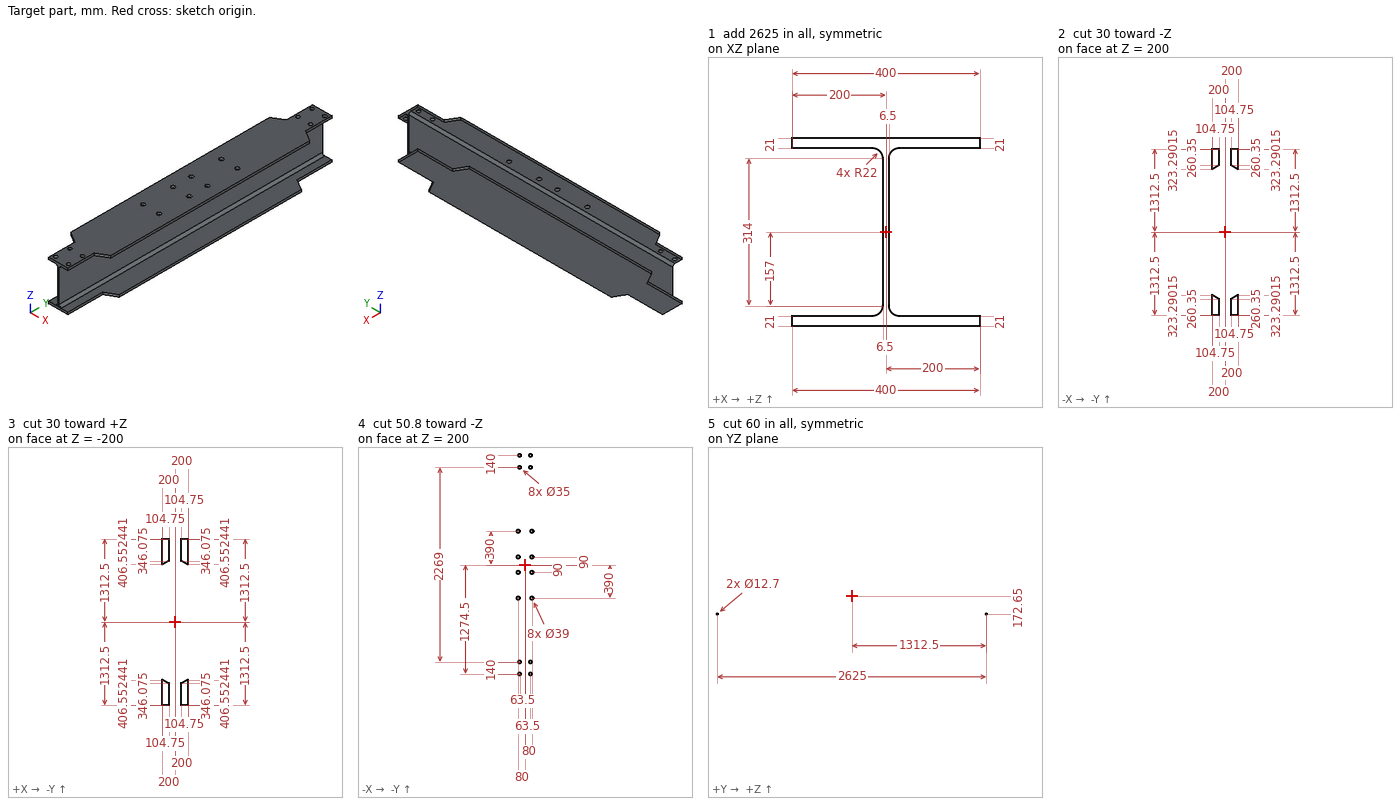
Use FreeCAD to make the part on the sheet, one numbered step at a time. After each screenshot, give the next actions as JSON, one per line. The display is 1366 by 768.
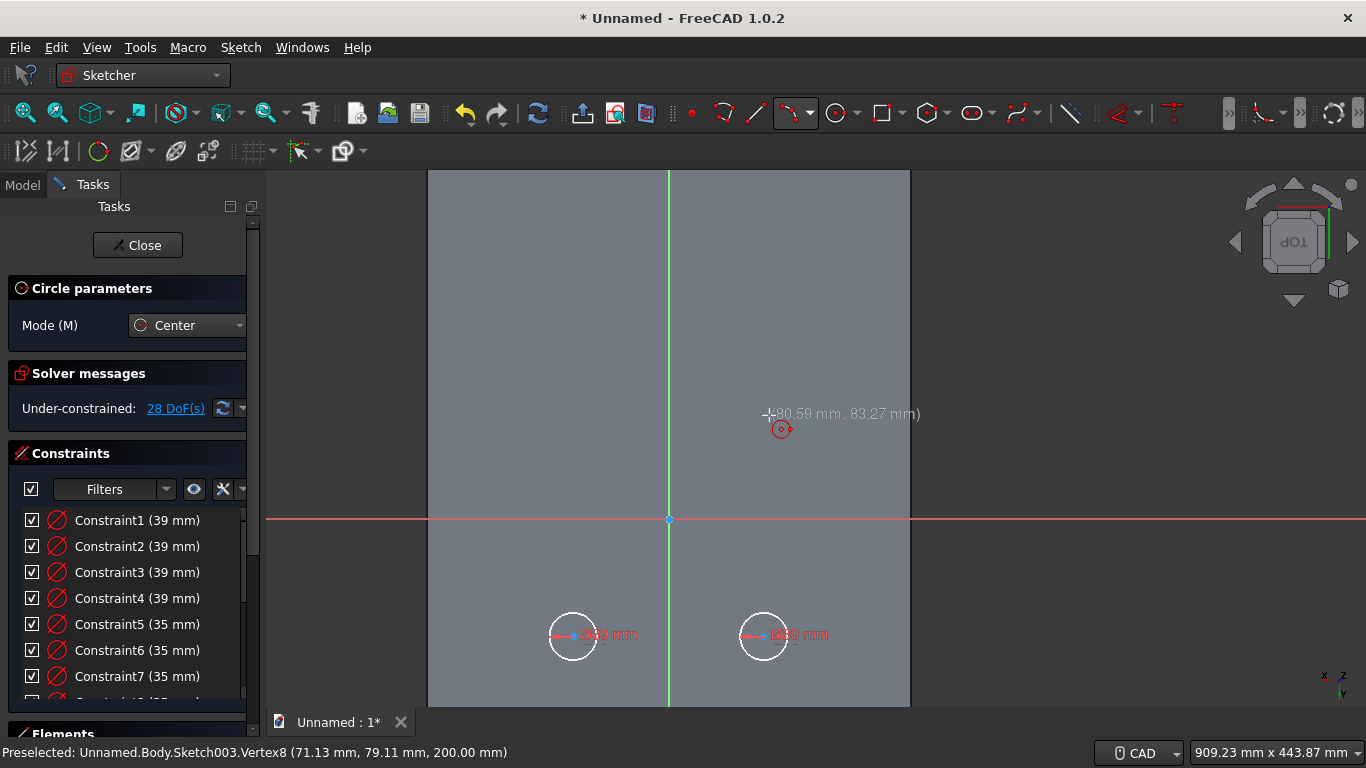
{"action": "scroll", "coordinate": [757, 428], "scroll_direction": "down", "scroll_amount": 11}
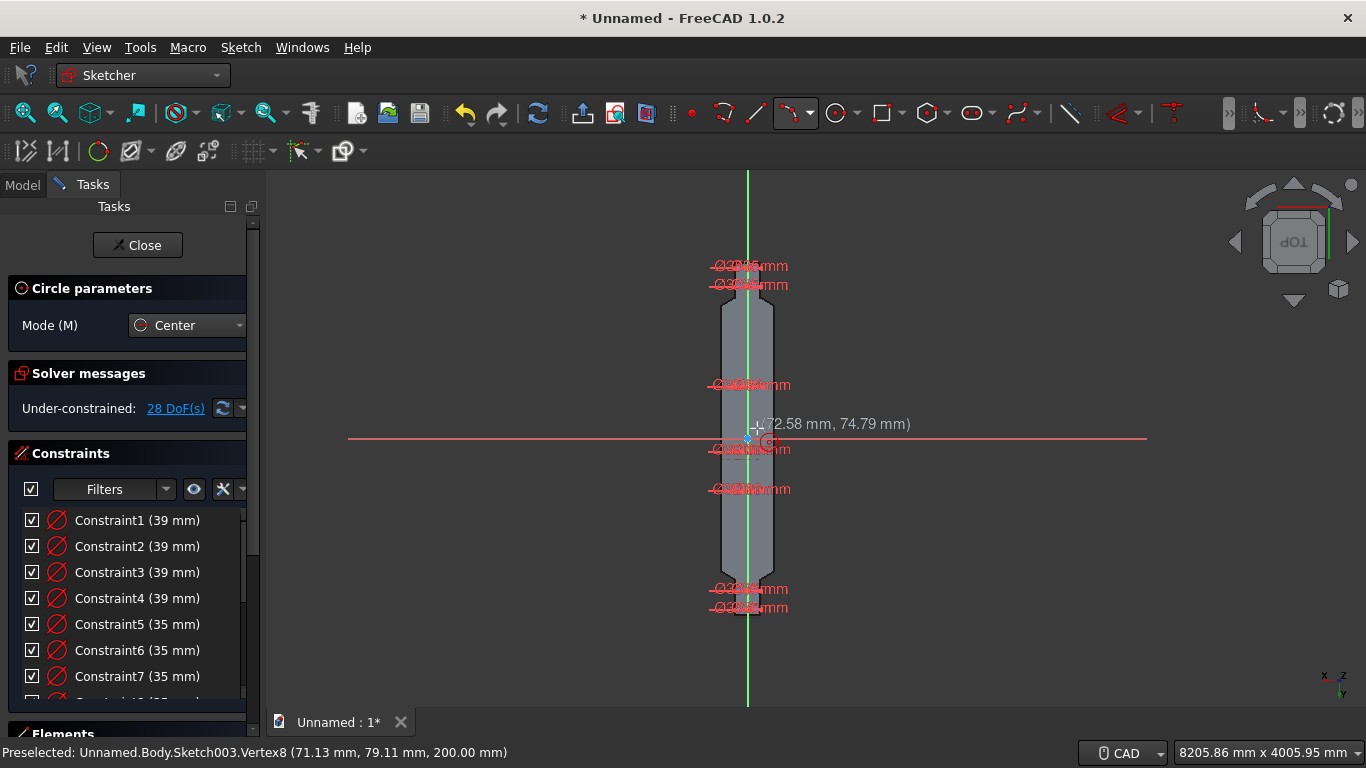
{"action": "scroll", "coordinate": [758, 426], "scroll_direction": "up", "scroll_amount": 2}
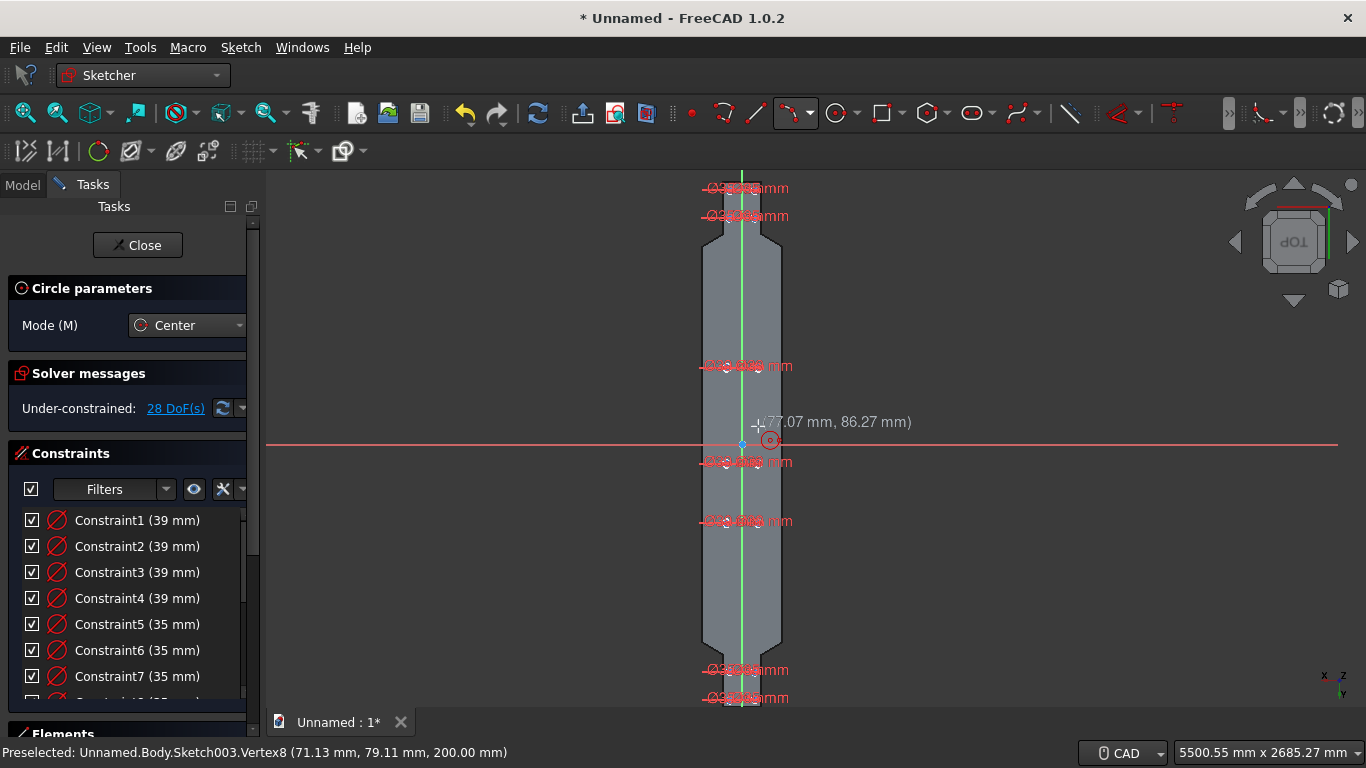
{"action": "left_click", "coordinate": [758, 427]}
{"action": "mouse_move", "coordinate": [761, 424]}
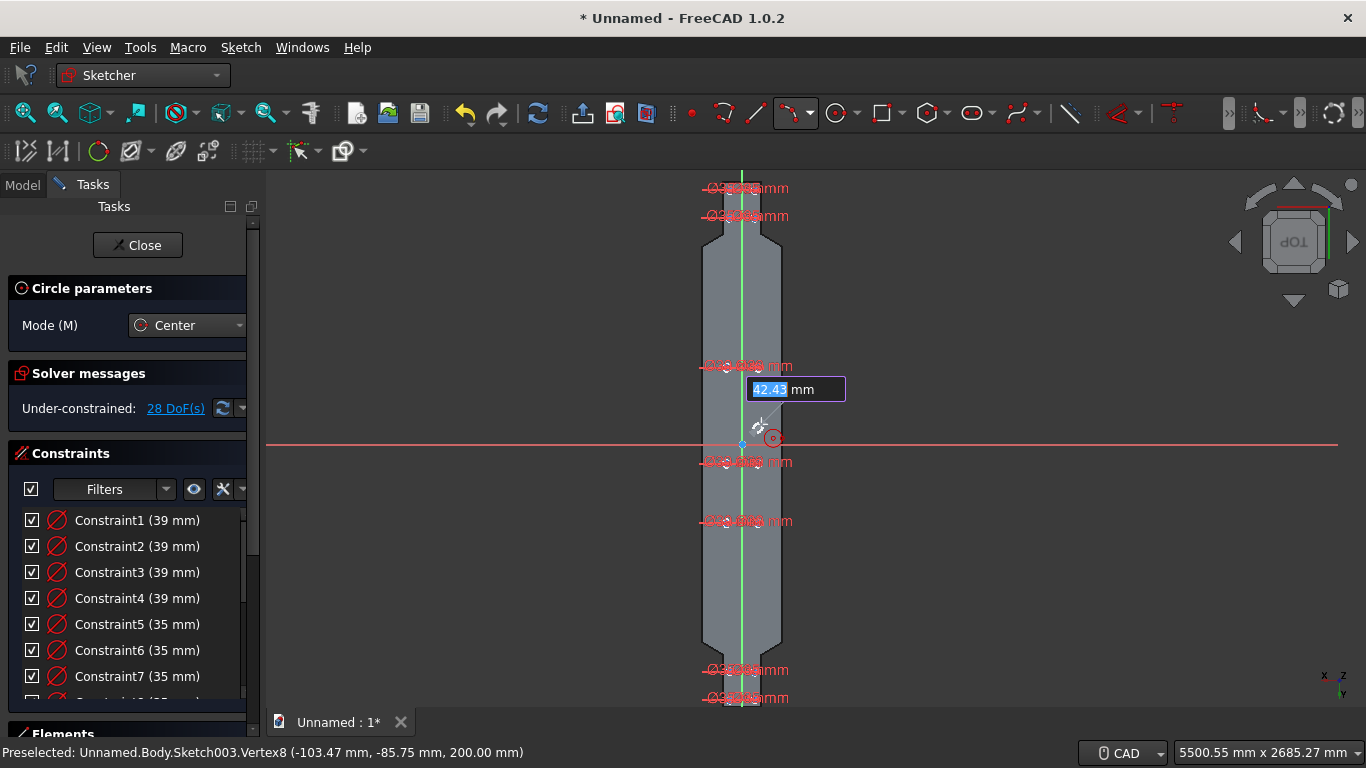
{"action": "type", "text": "39"}
{"action": "key", "text": "Return"}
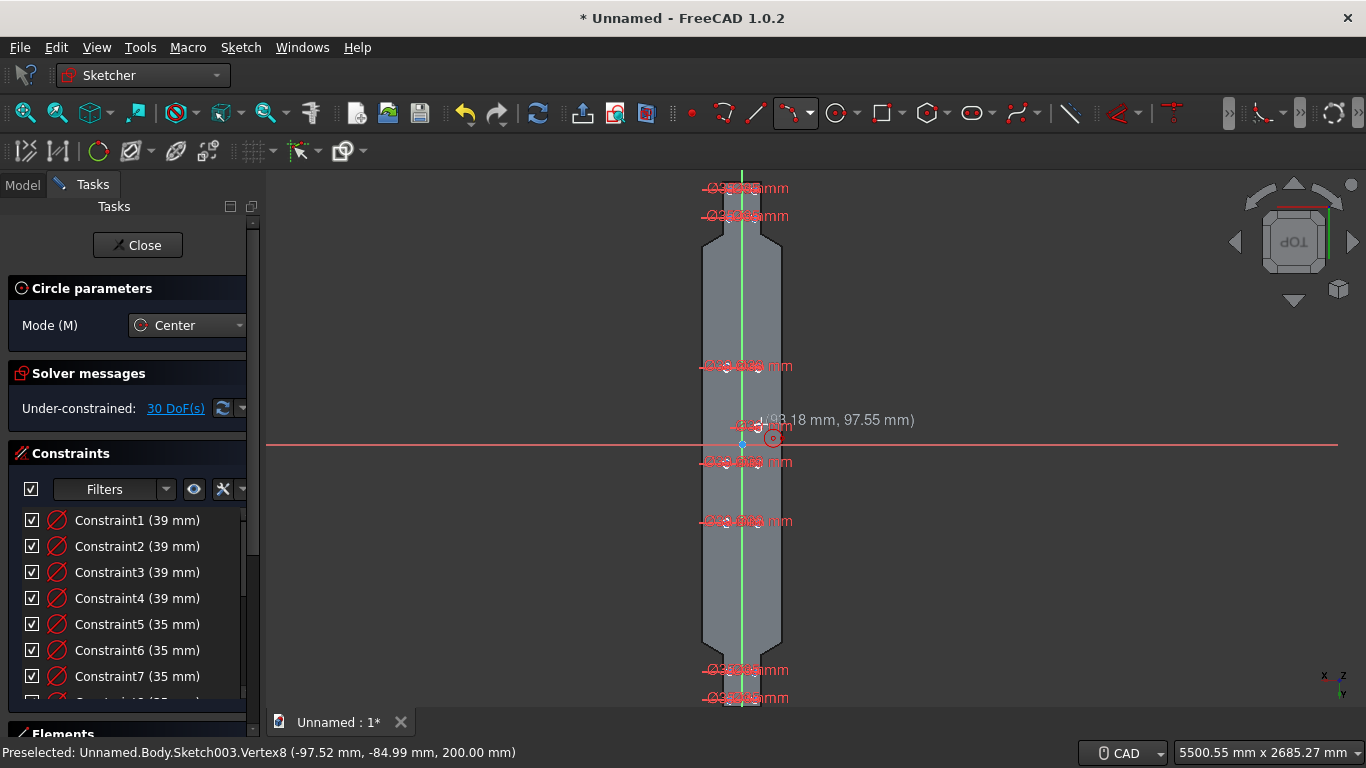
{"action": "scroll", "coordinate": [726, 427], "scroll_direction": "up", "scroll_amount": 9}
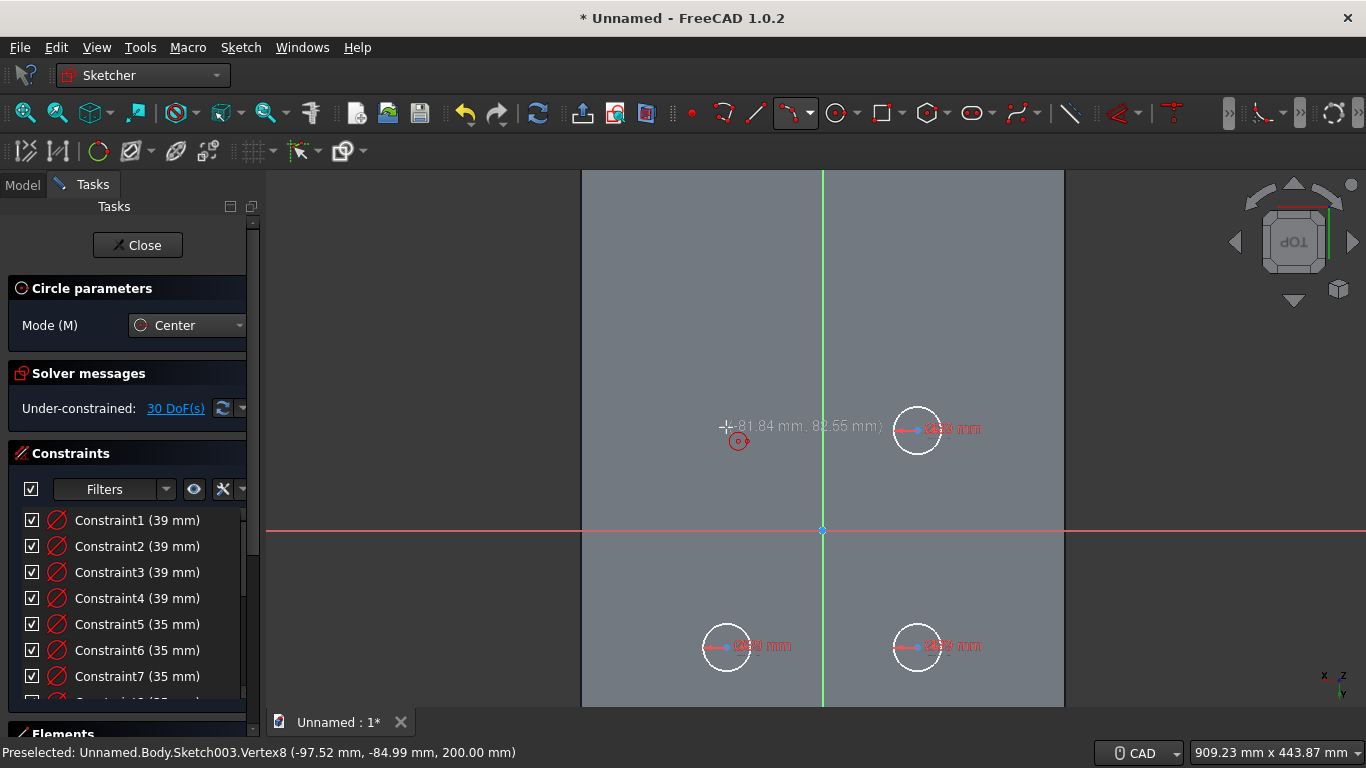
{"action": "scroll", "coordinate": [738, 427], "scroll_direction": "down", "scroll_amount": 11}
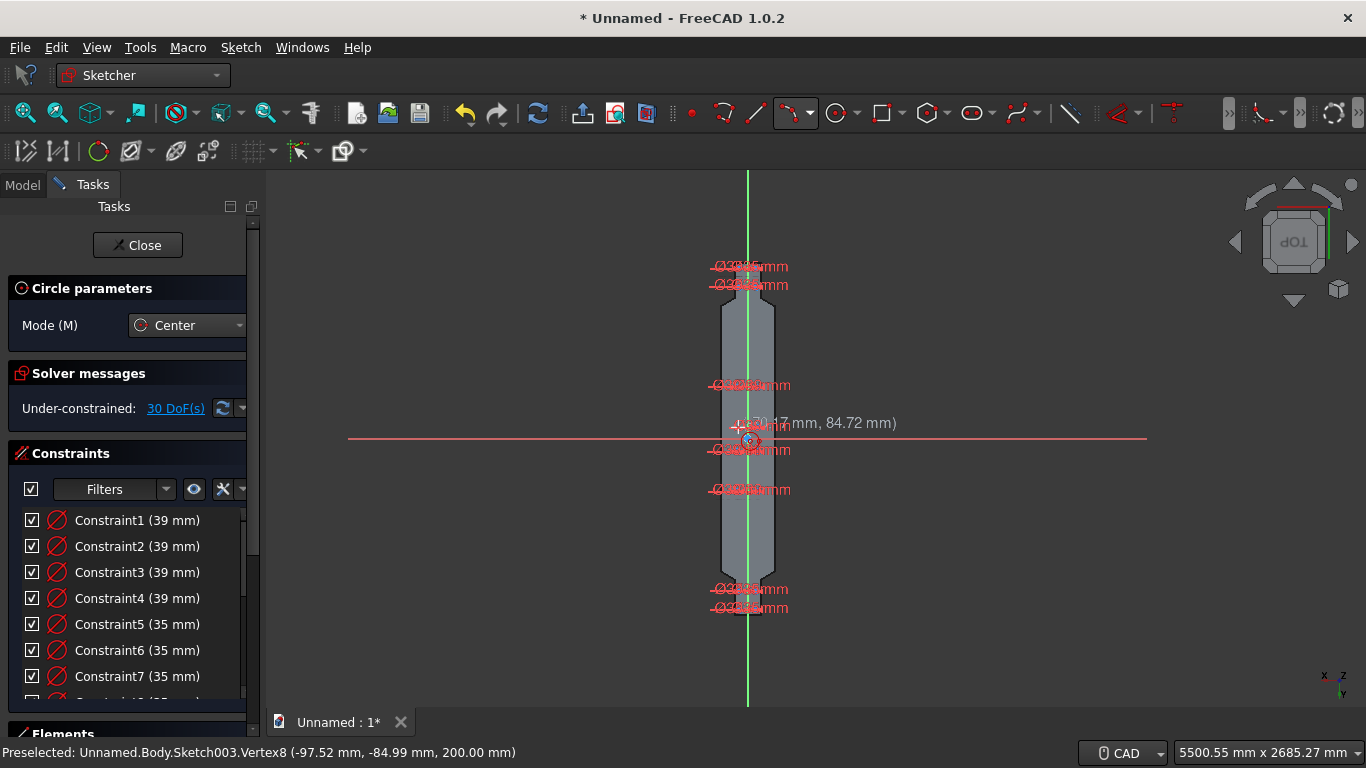
{"action": "scroll", "coordinate": [737, 427], "scroll_direction": "up", "scroll_amount": 2}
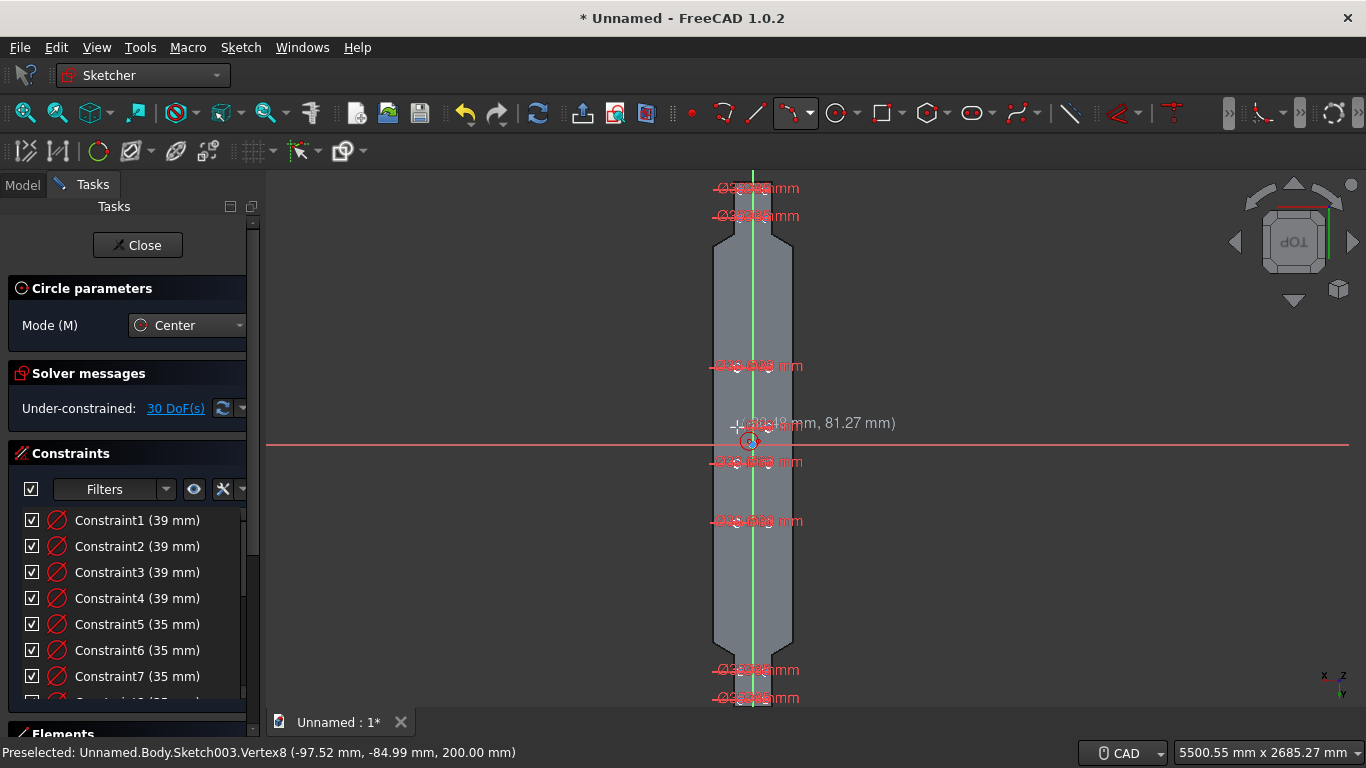
{"action": "left_click", "coordinate": [737, 427]}
{"action": "mouse_move", "coordinate": [734, 424]}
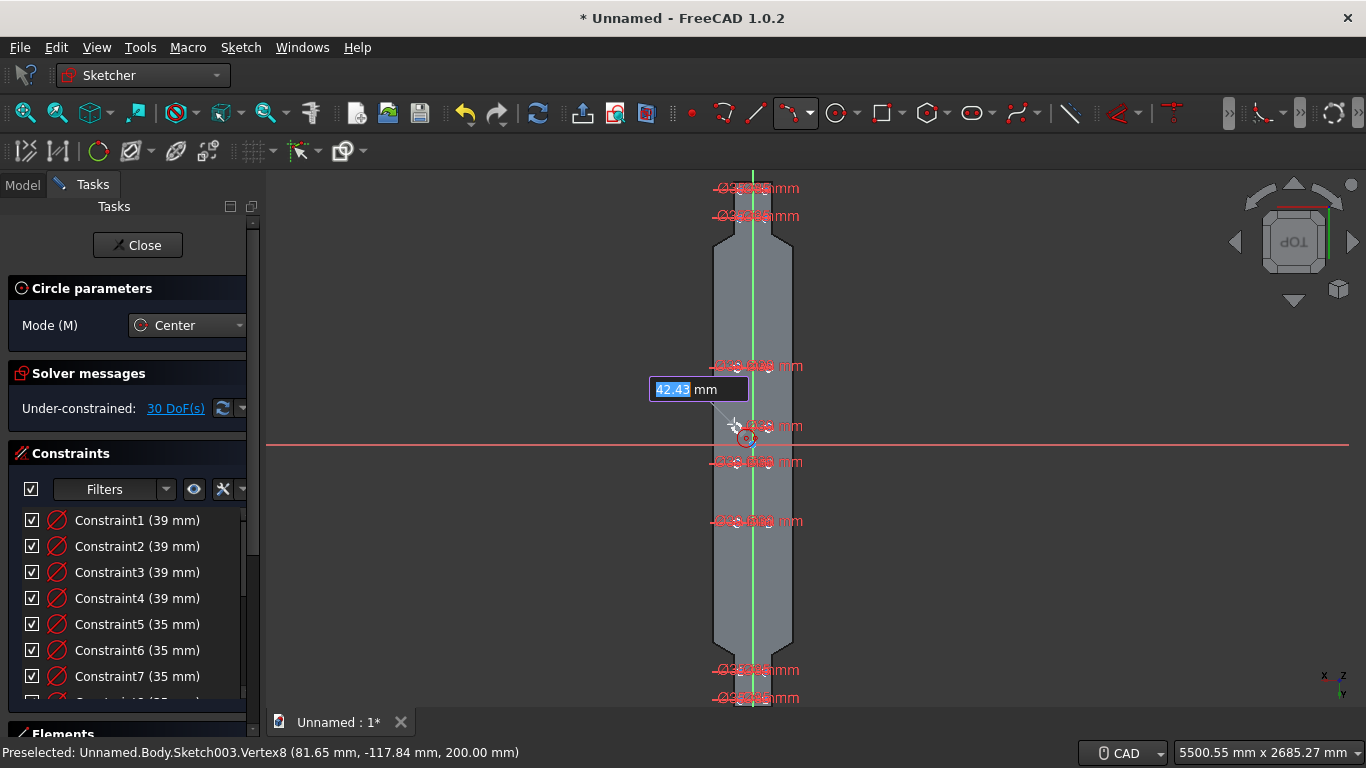
{"action": "type", "text": "39"}
{"action": "key", "text": "Return"}
{"action": "key", "text": "Escape"}